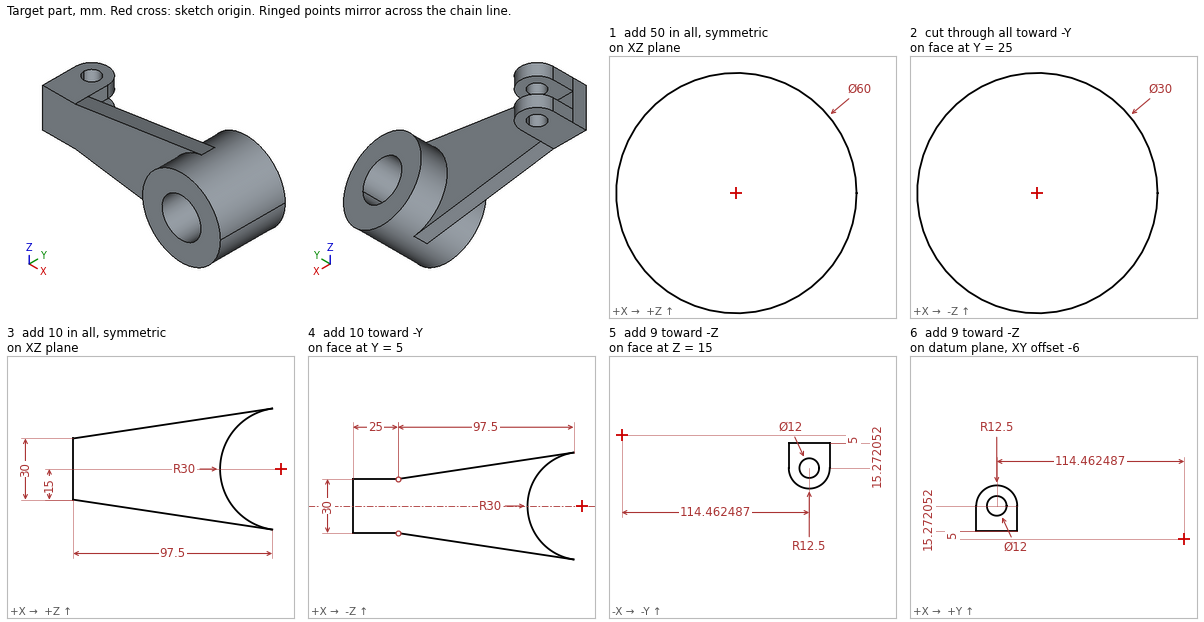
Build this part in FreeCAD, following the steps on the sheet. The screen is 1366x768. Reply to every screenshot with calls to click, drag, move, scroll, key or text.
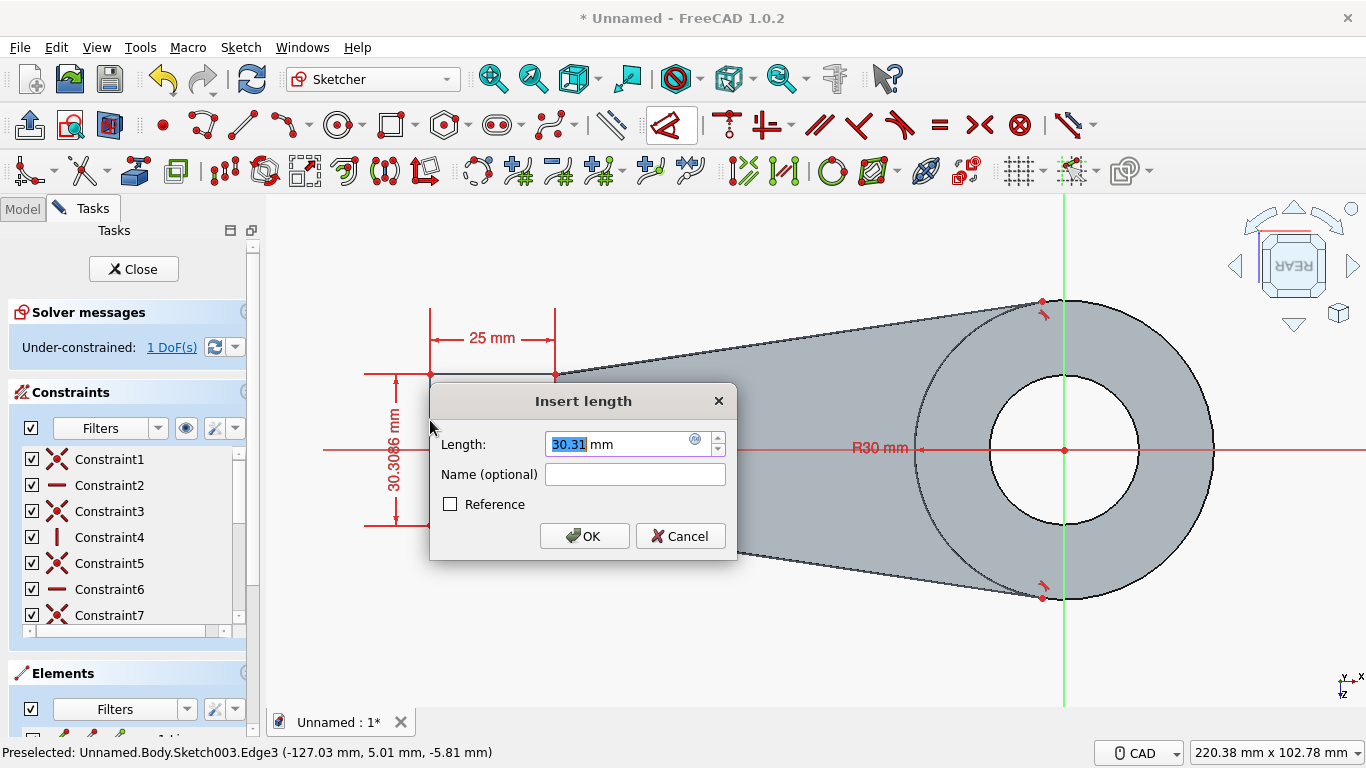
text(30)
key(Return)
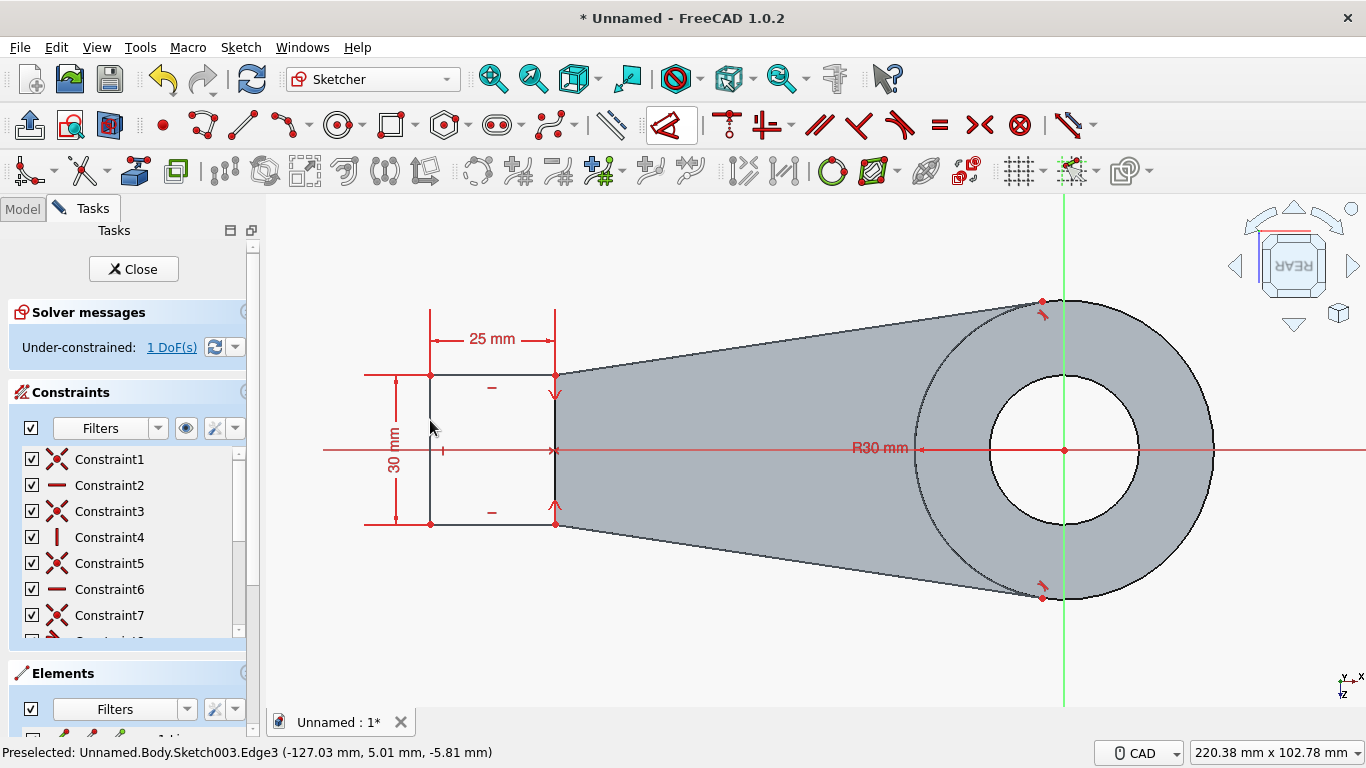
click(896, 324)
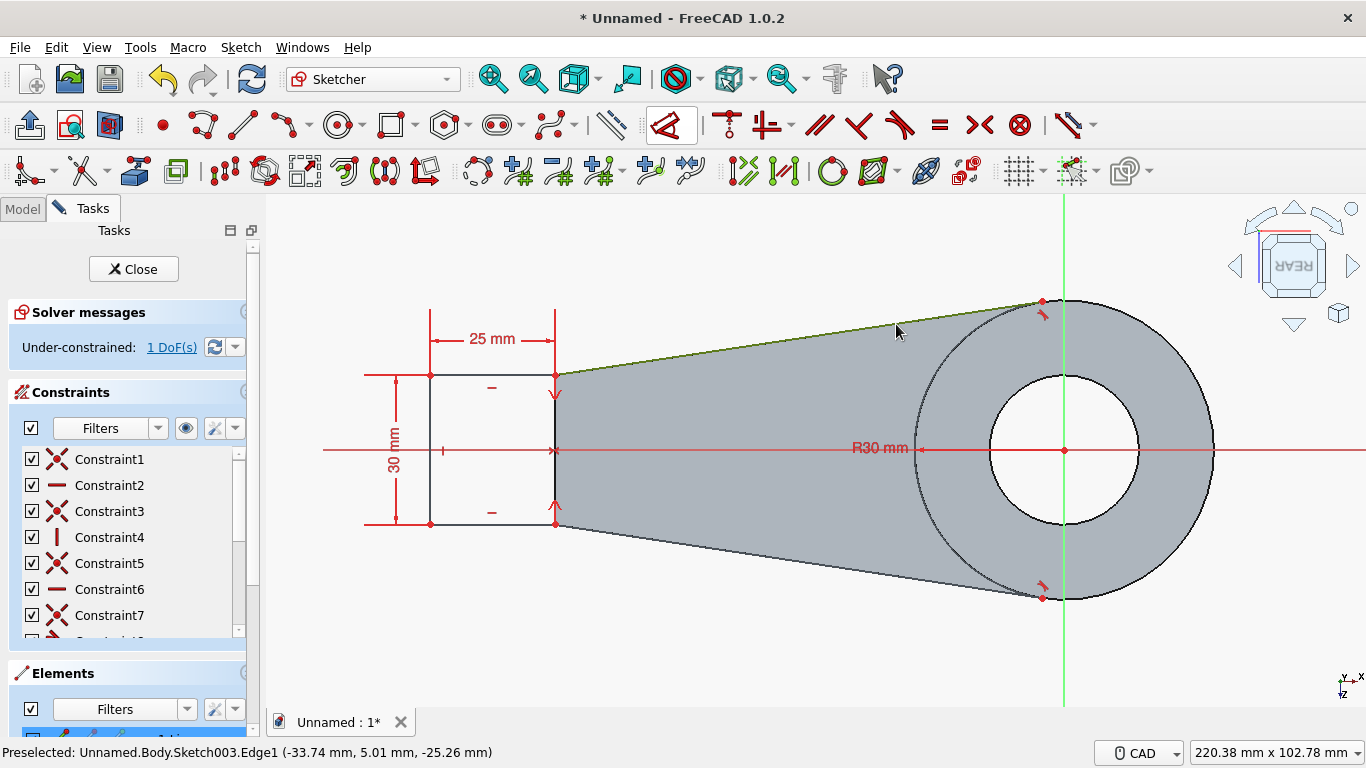
click(692, 126)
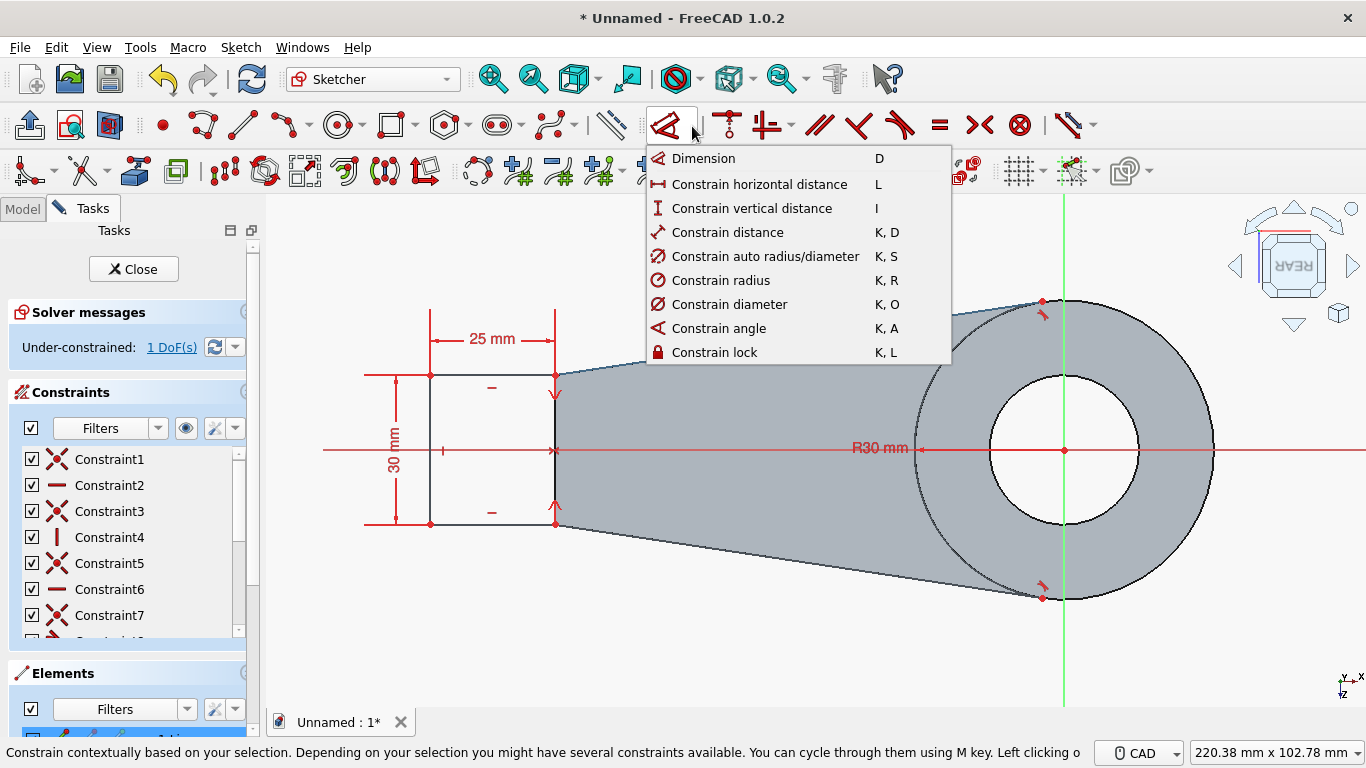
click(799, 184)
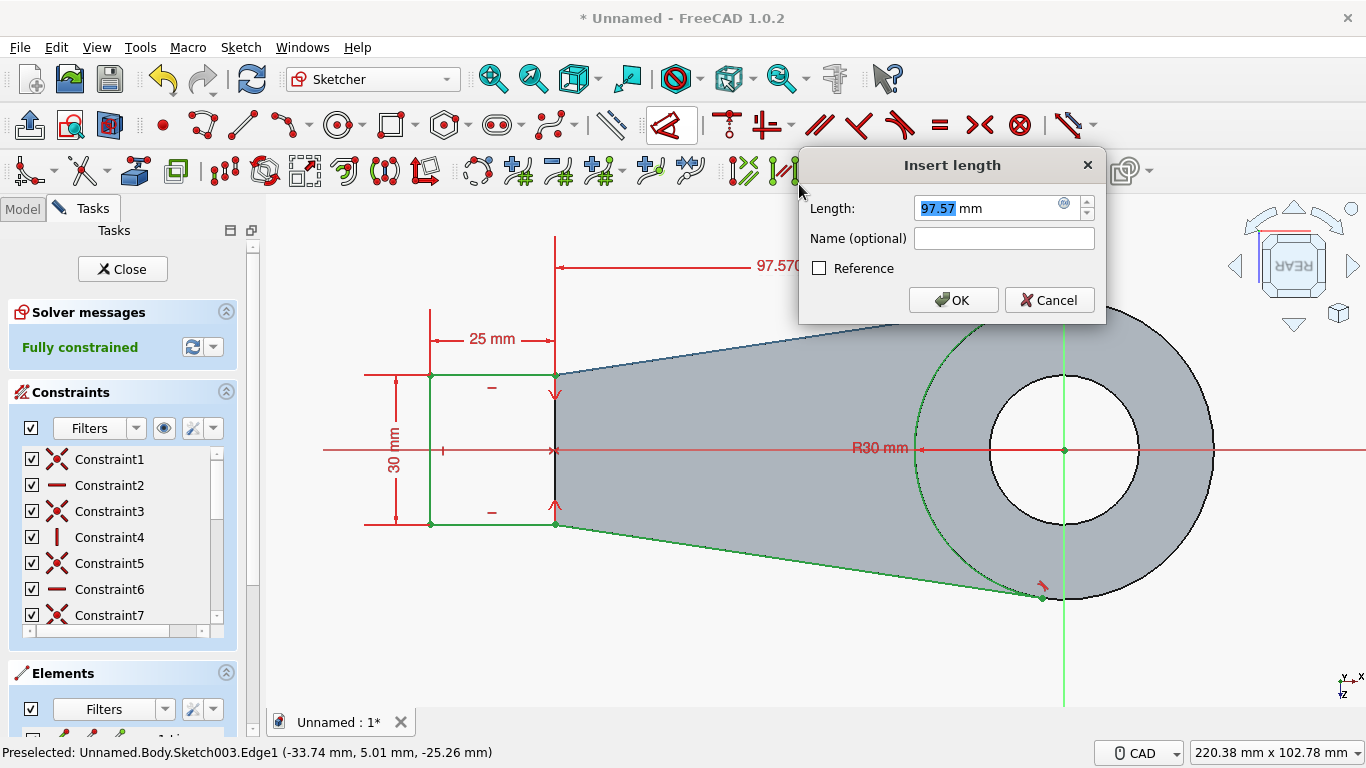
text(97.5)
key(Return)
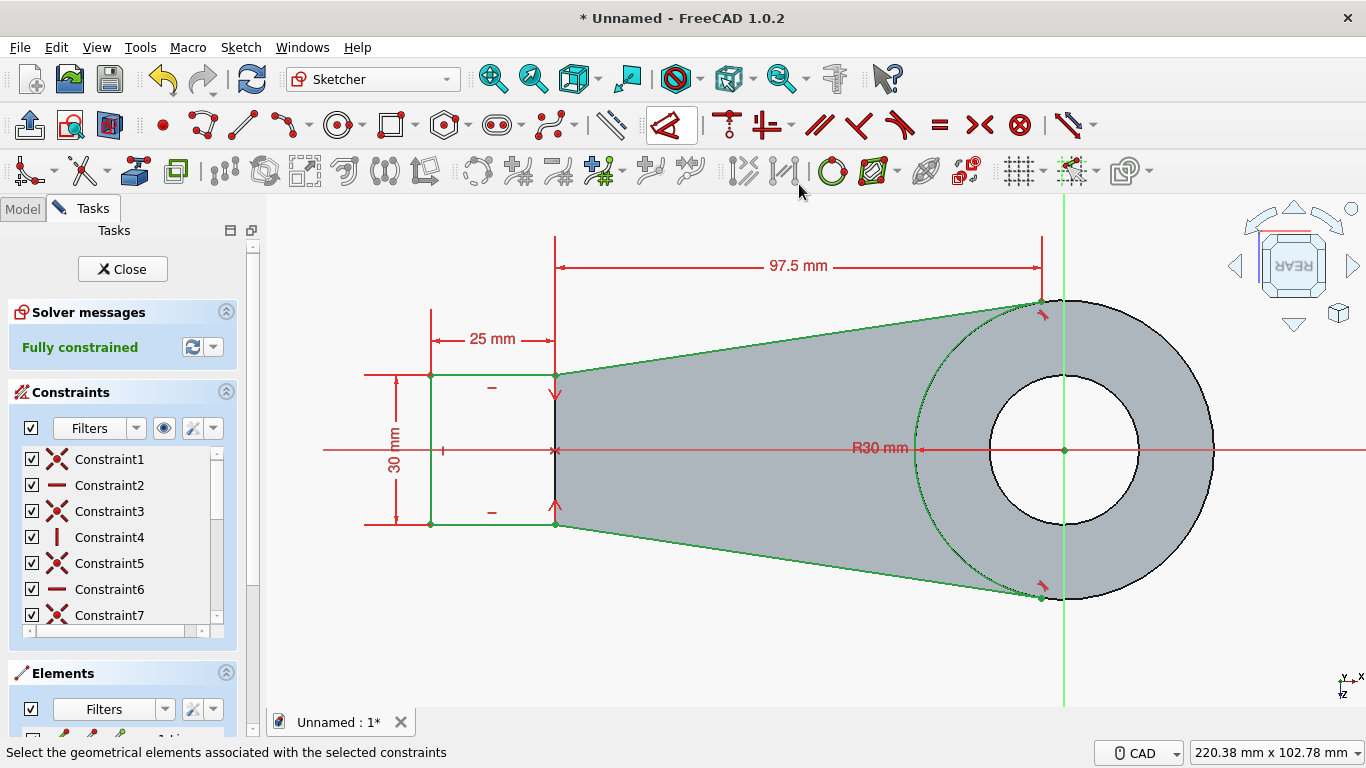
click(123, 269)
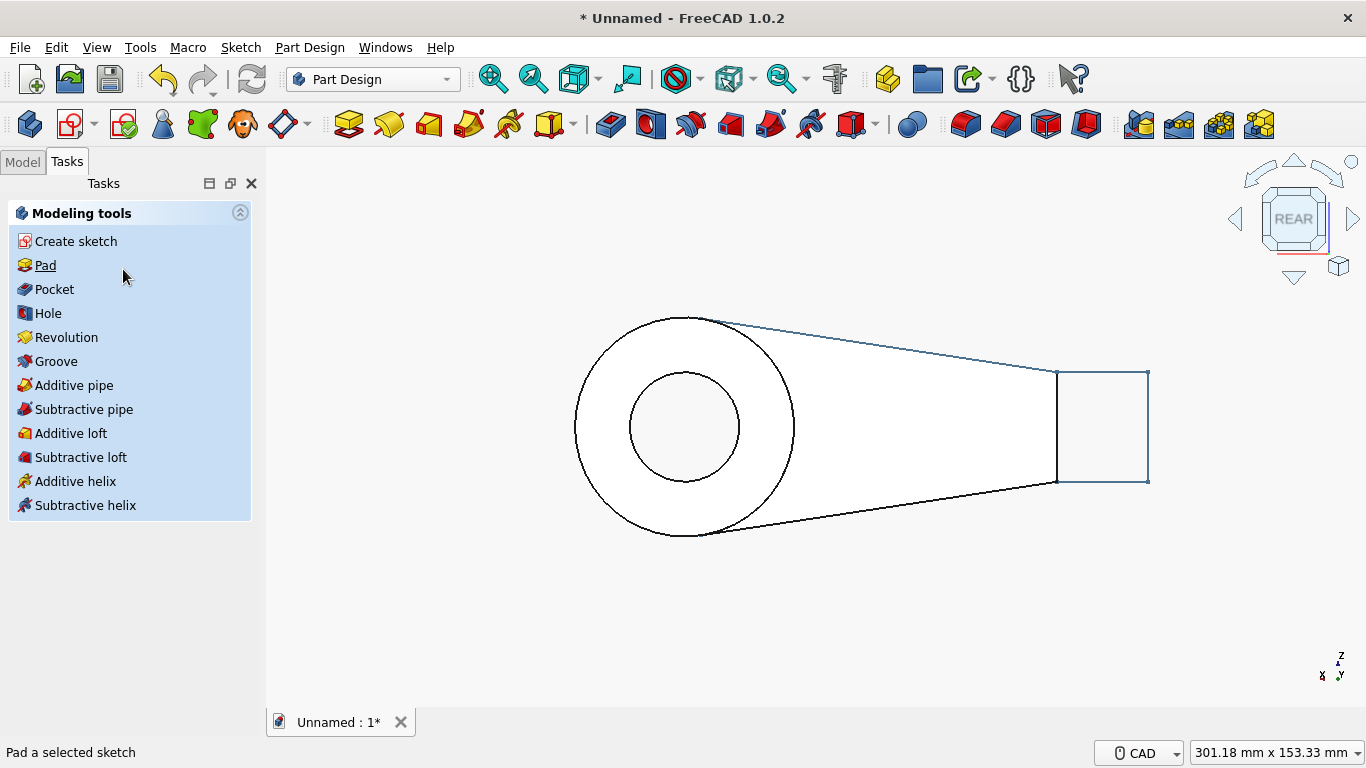
click(350, 124)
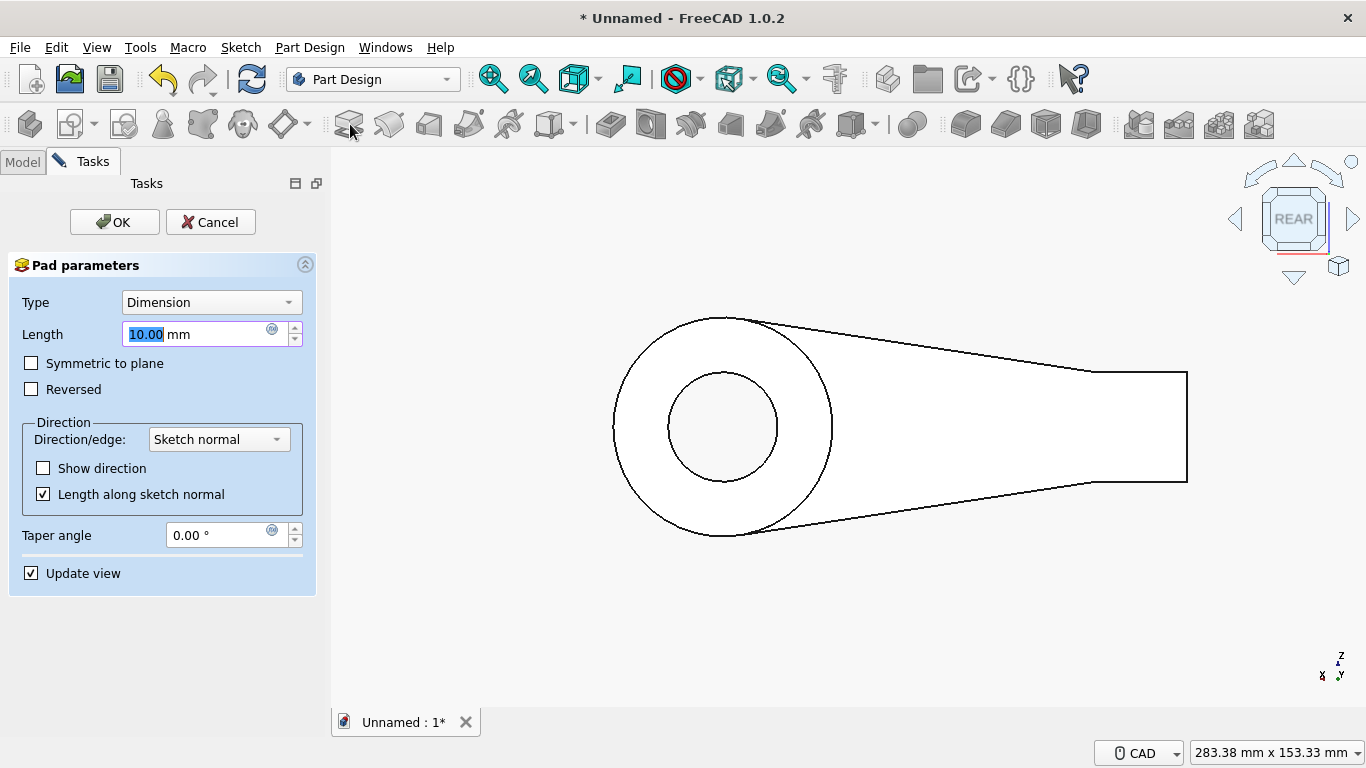
text(10)
key(Tab)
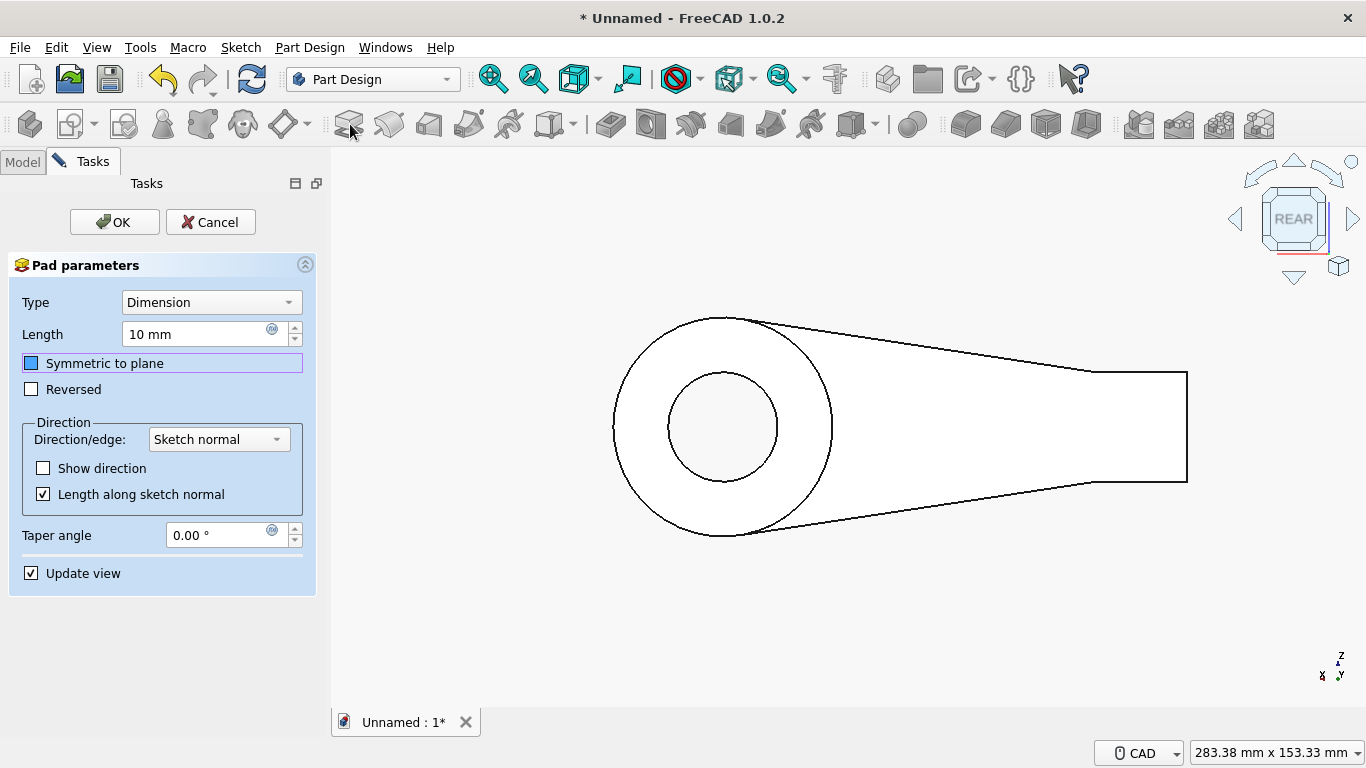
click(30, 389)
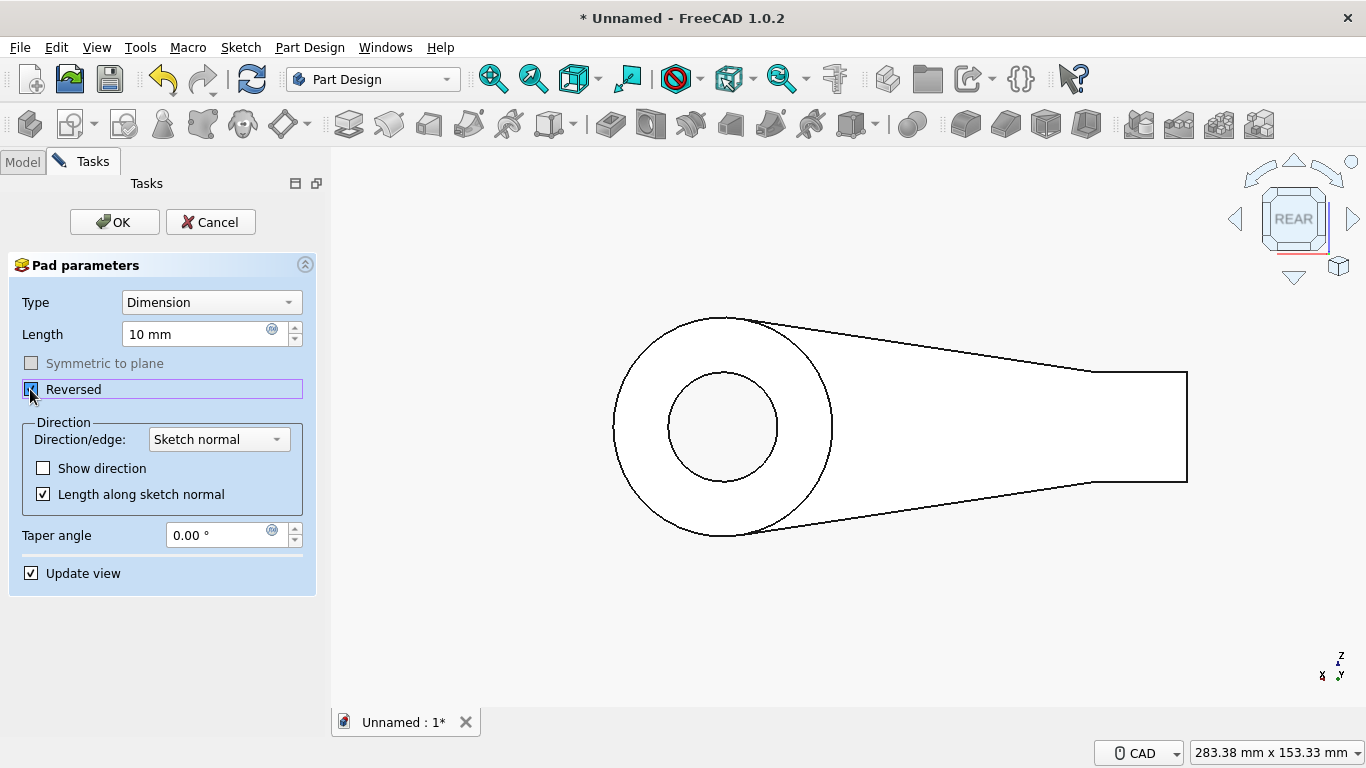
click(115, 222)